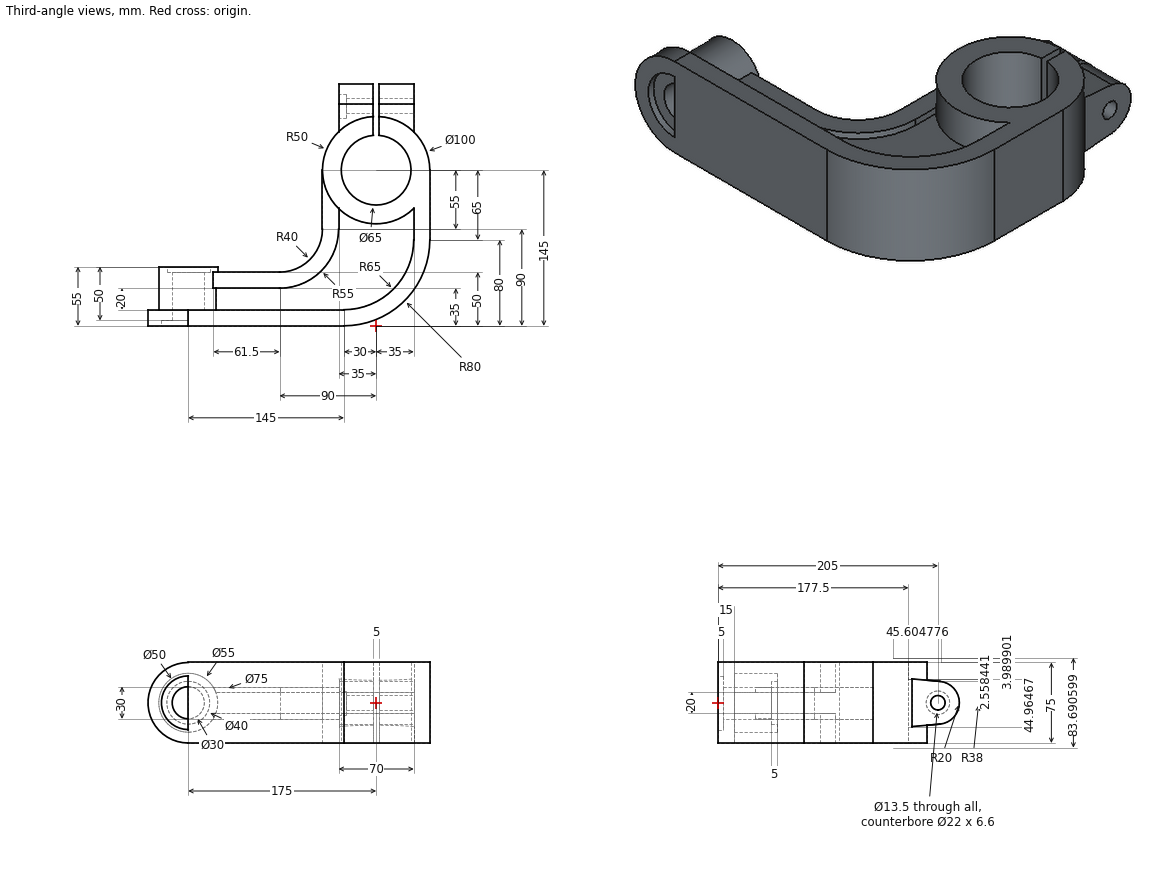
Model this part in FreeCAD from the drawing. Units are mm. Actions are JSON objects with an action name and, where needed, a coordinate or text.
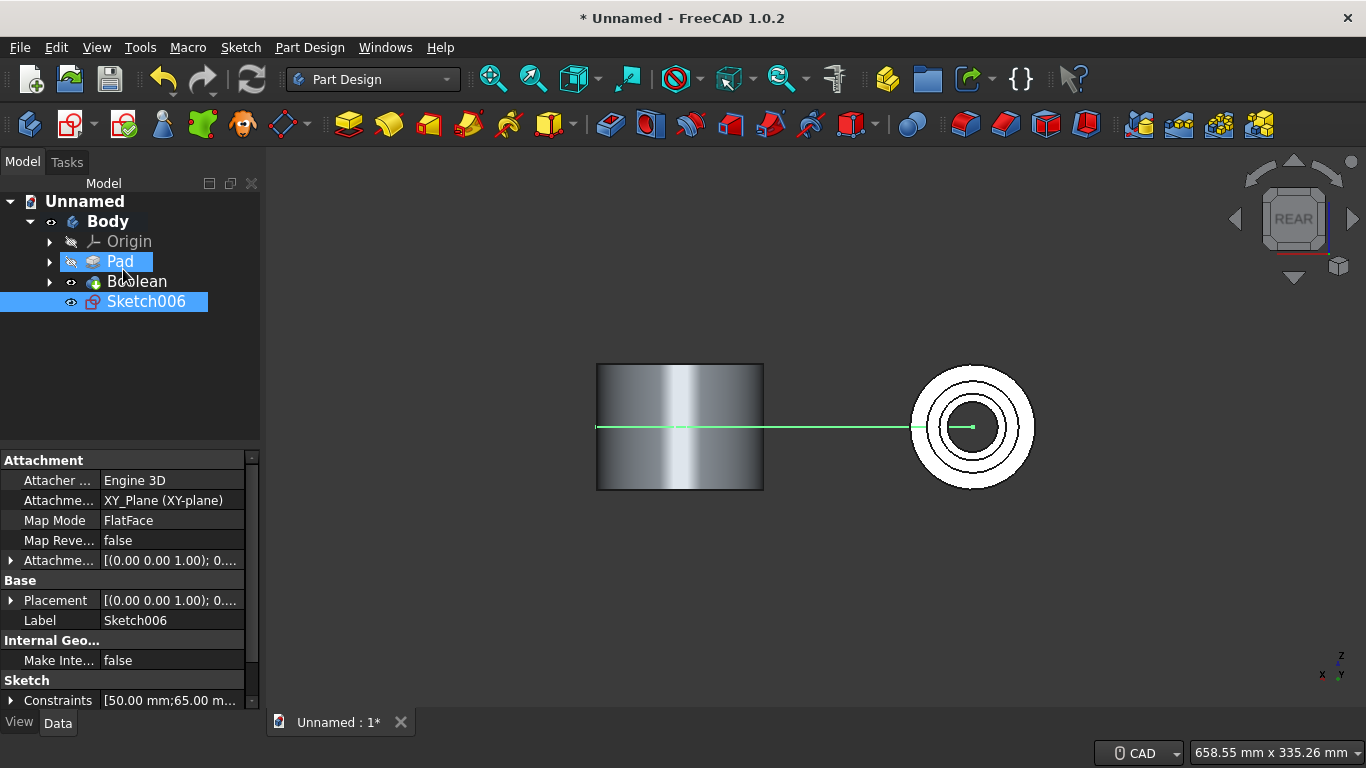
{"action": "left_click", "coordinate": [350, 124]}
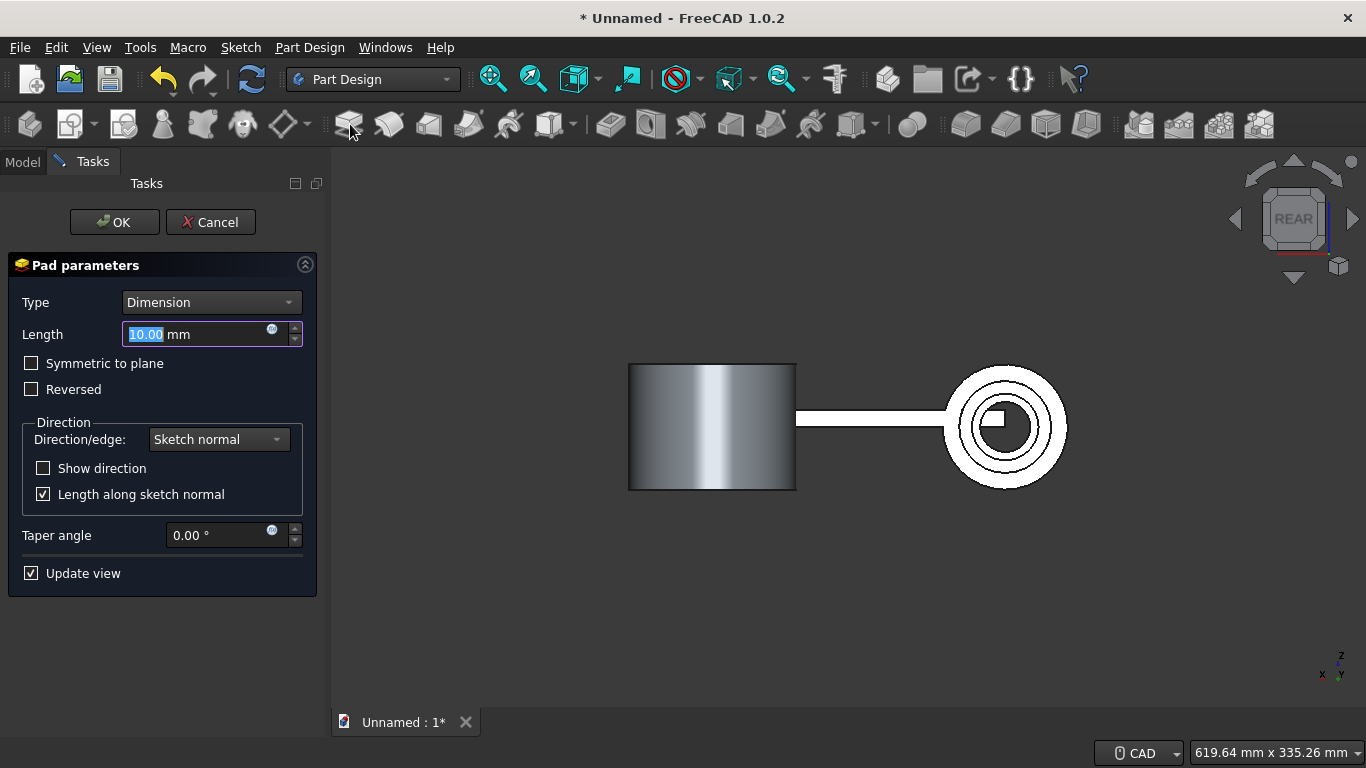
{"action": "type", "text": "75"}
{"action": "key", "text": "Tab"}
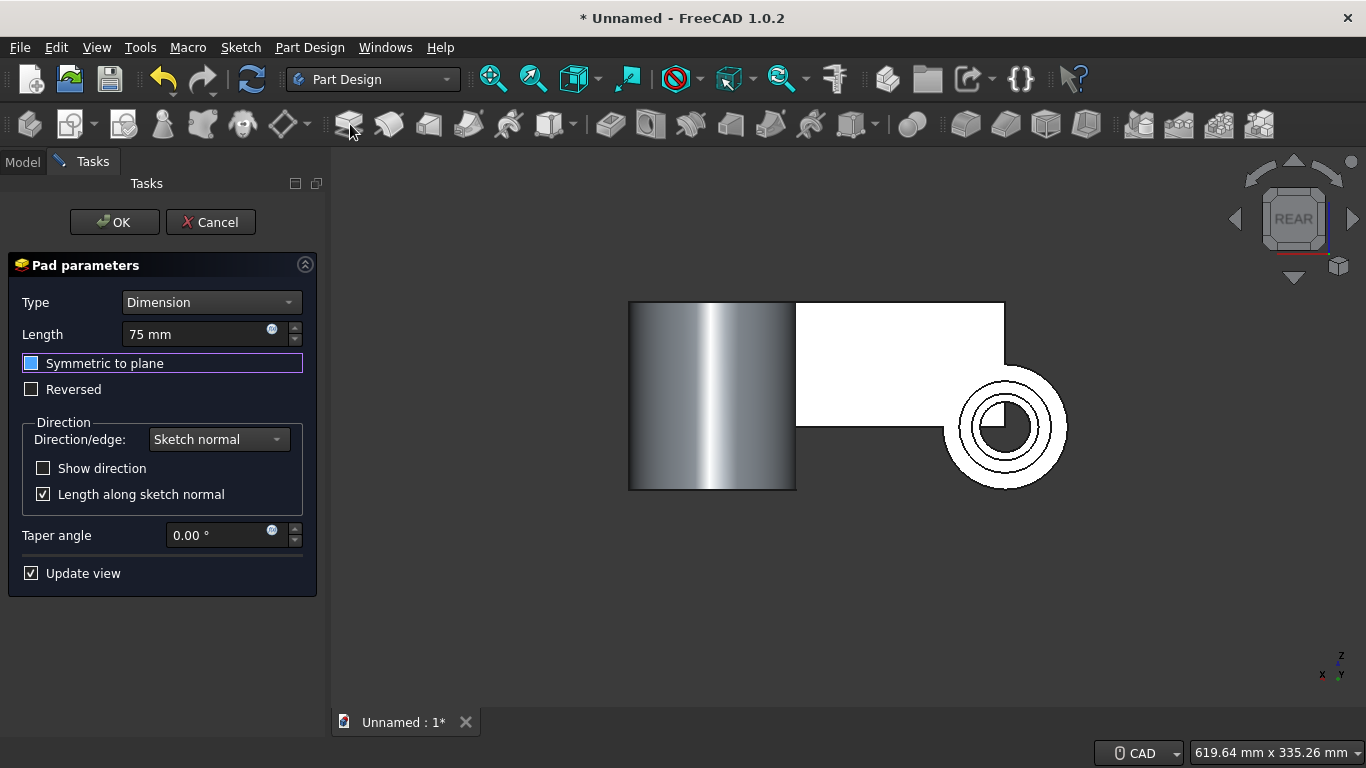
{"action": "left_click", "coordinate": [30, 363]}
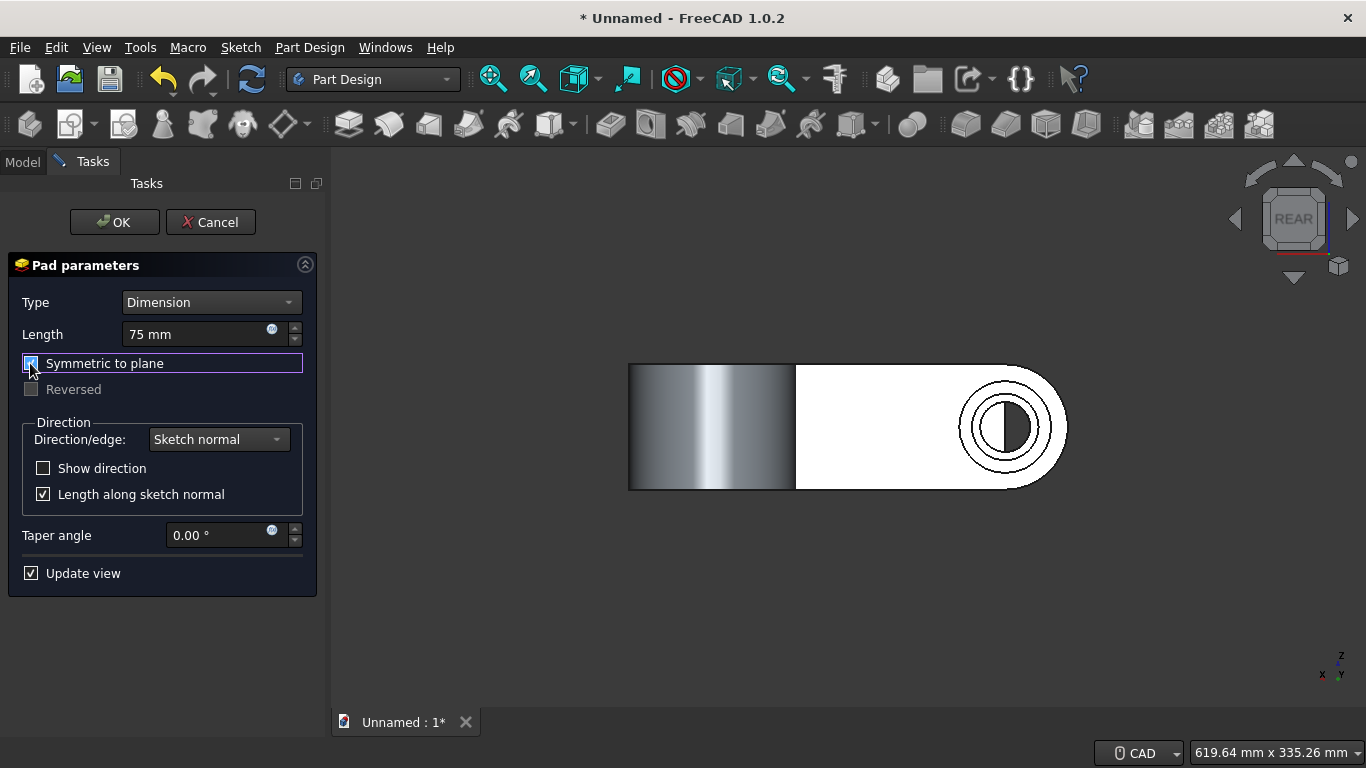
{"action": "left_click", "coordinate": [115, 222]}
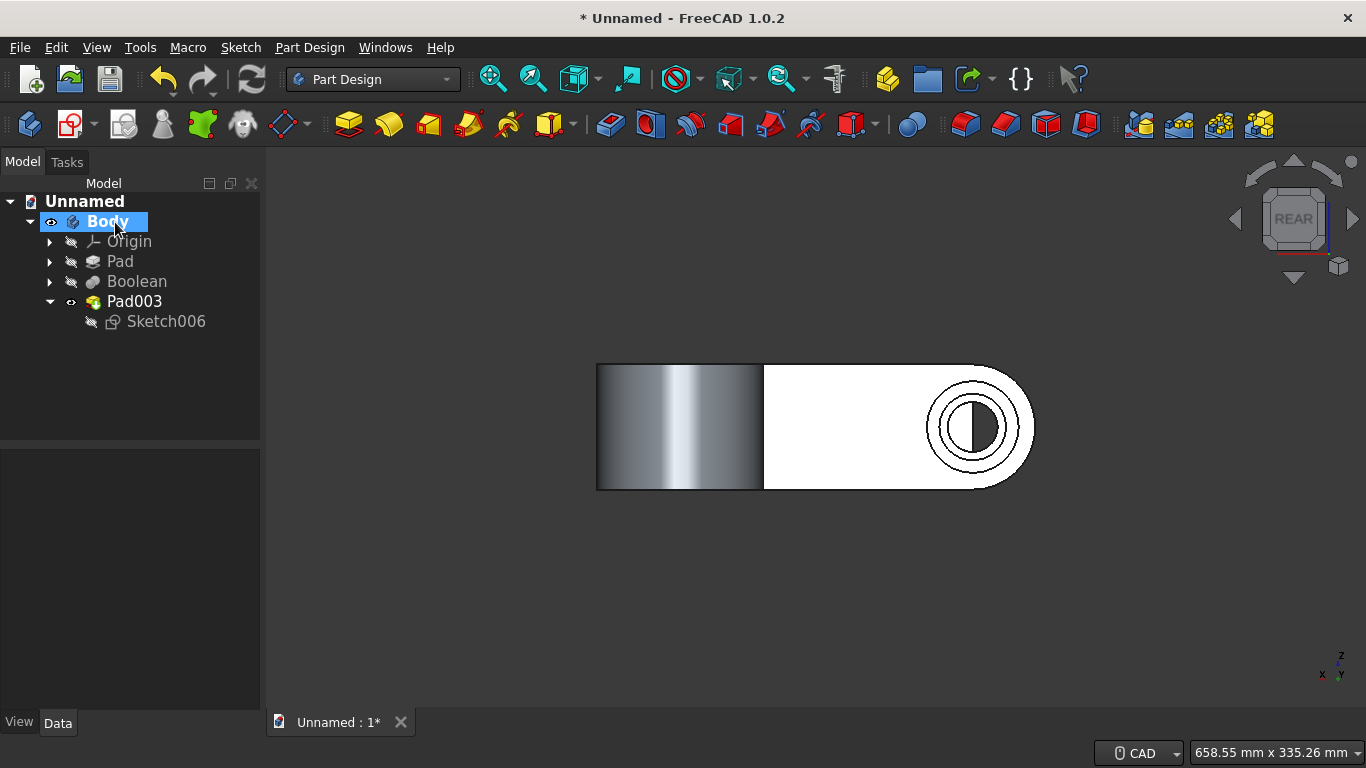
{"action": "key", "text": "v f"}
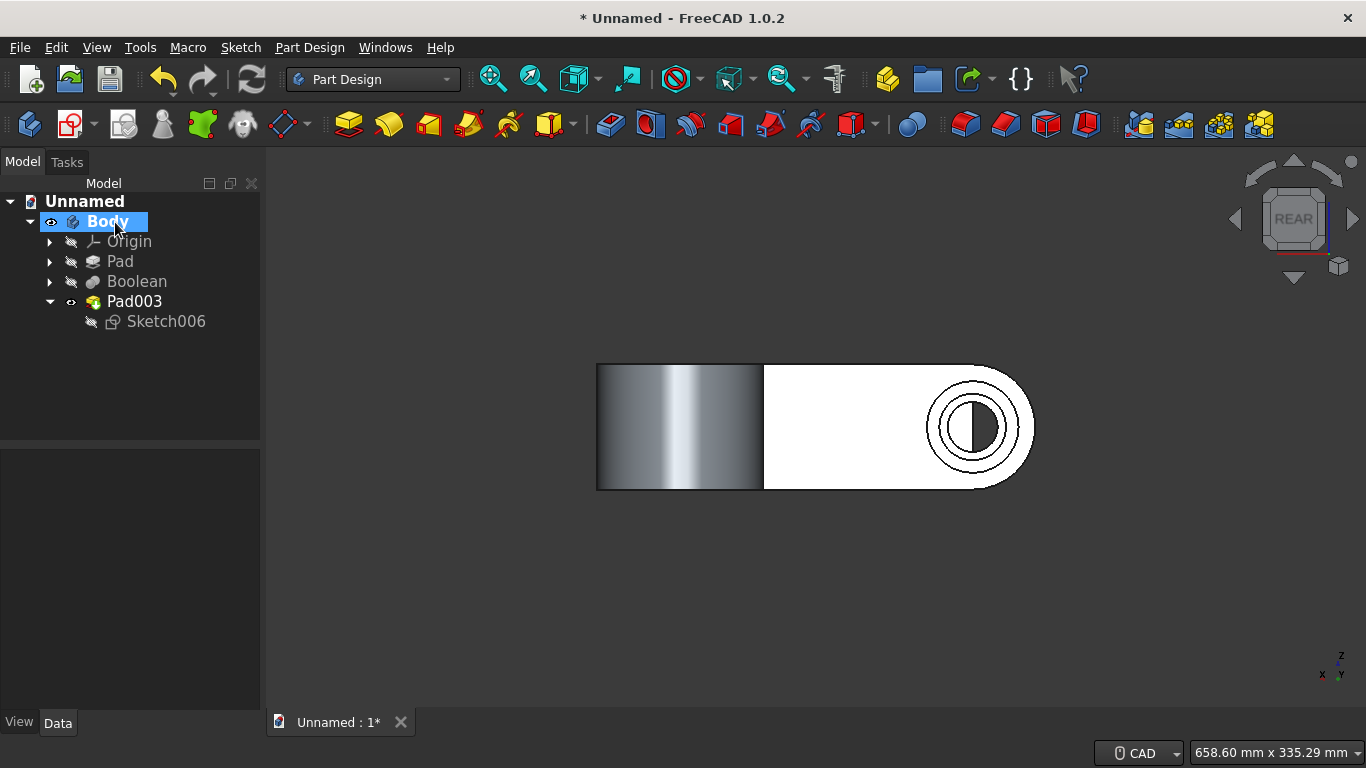
{"action": "left_click", "coordinate": [70, 124]}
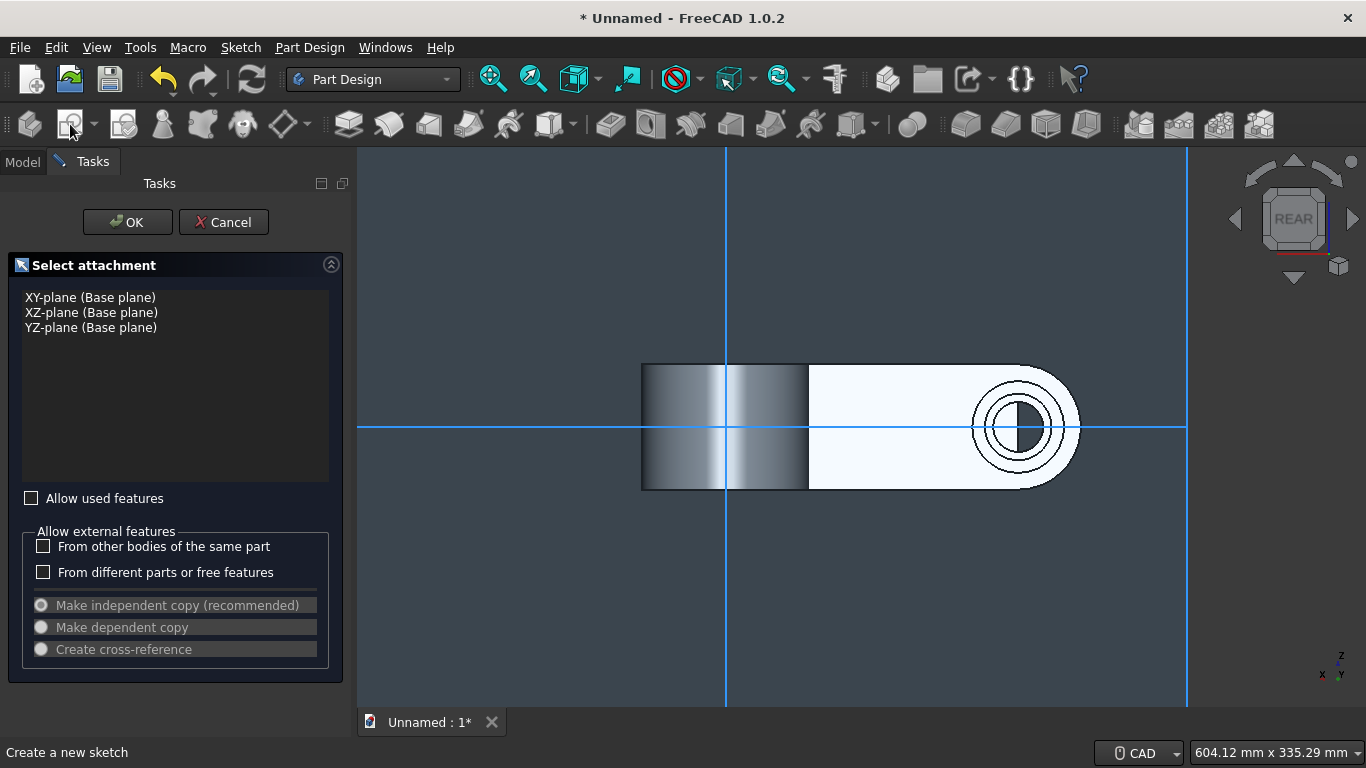
{"action": "left_click", "coordinate": [82, 298]}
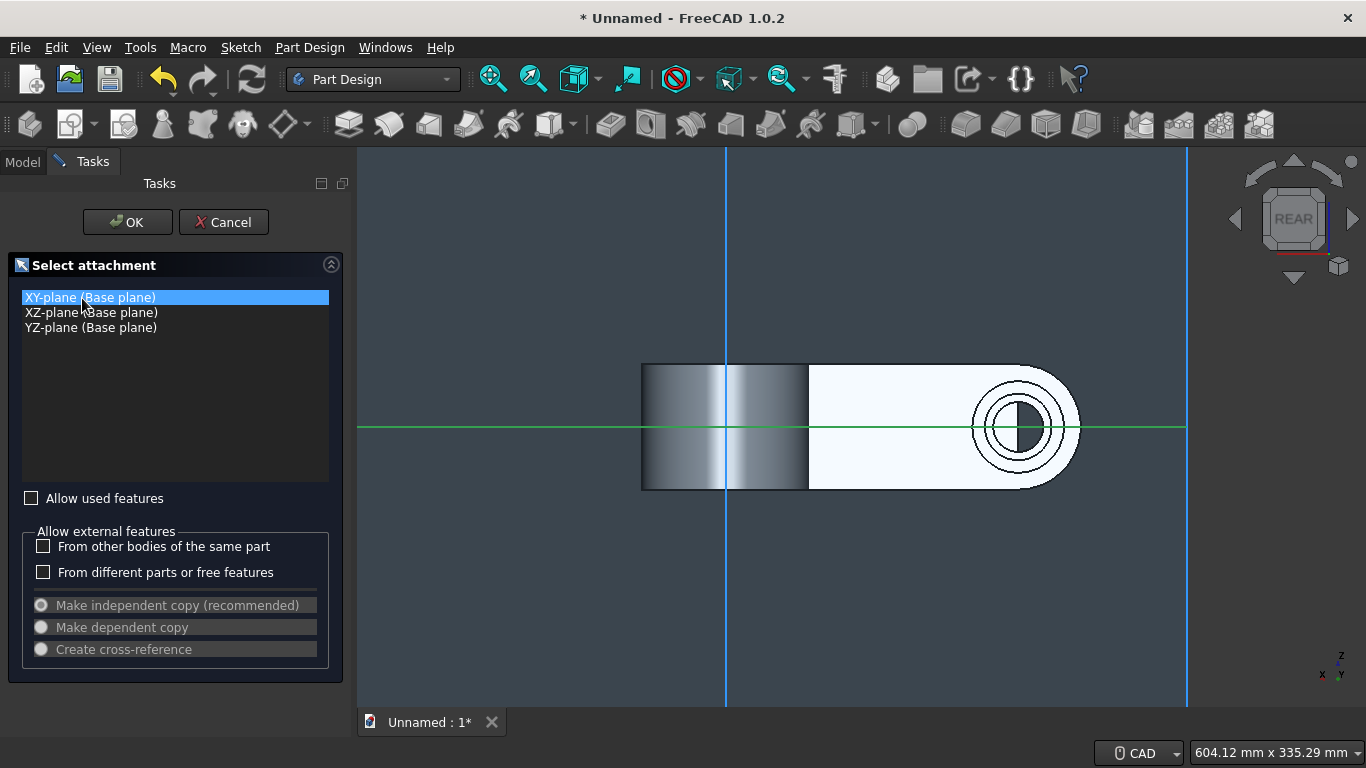
{"action": "left_click", "coordinate": [128, 222]}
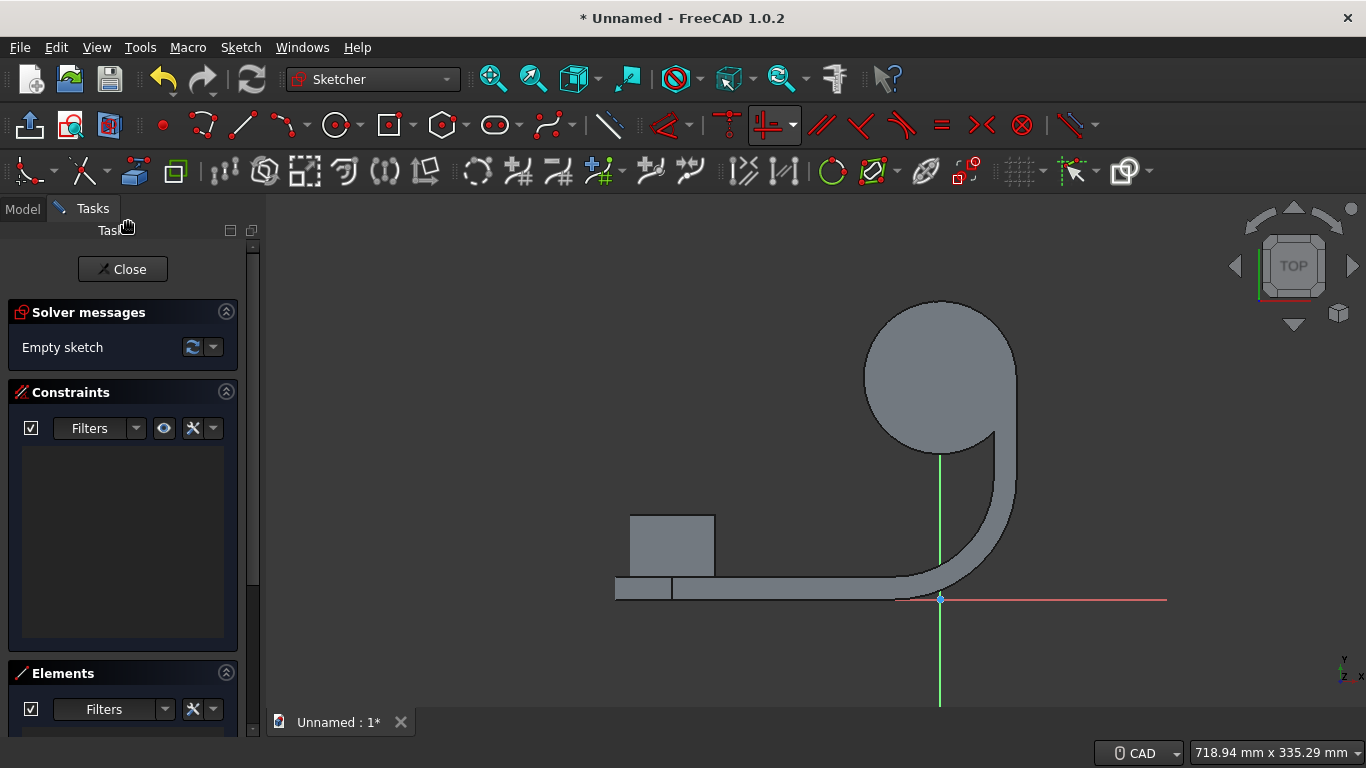
{"action": "left_click", "coordinate": [110, 126]}